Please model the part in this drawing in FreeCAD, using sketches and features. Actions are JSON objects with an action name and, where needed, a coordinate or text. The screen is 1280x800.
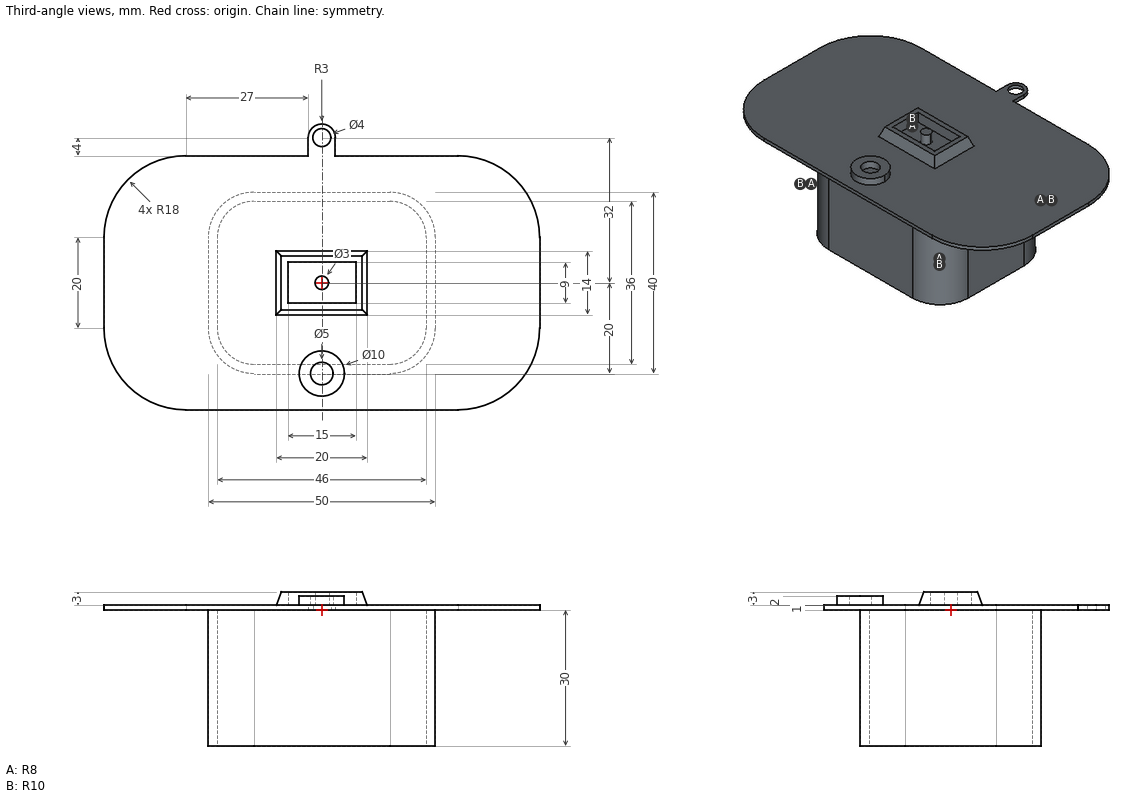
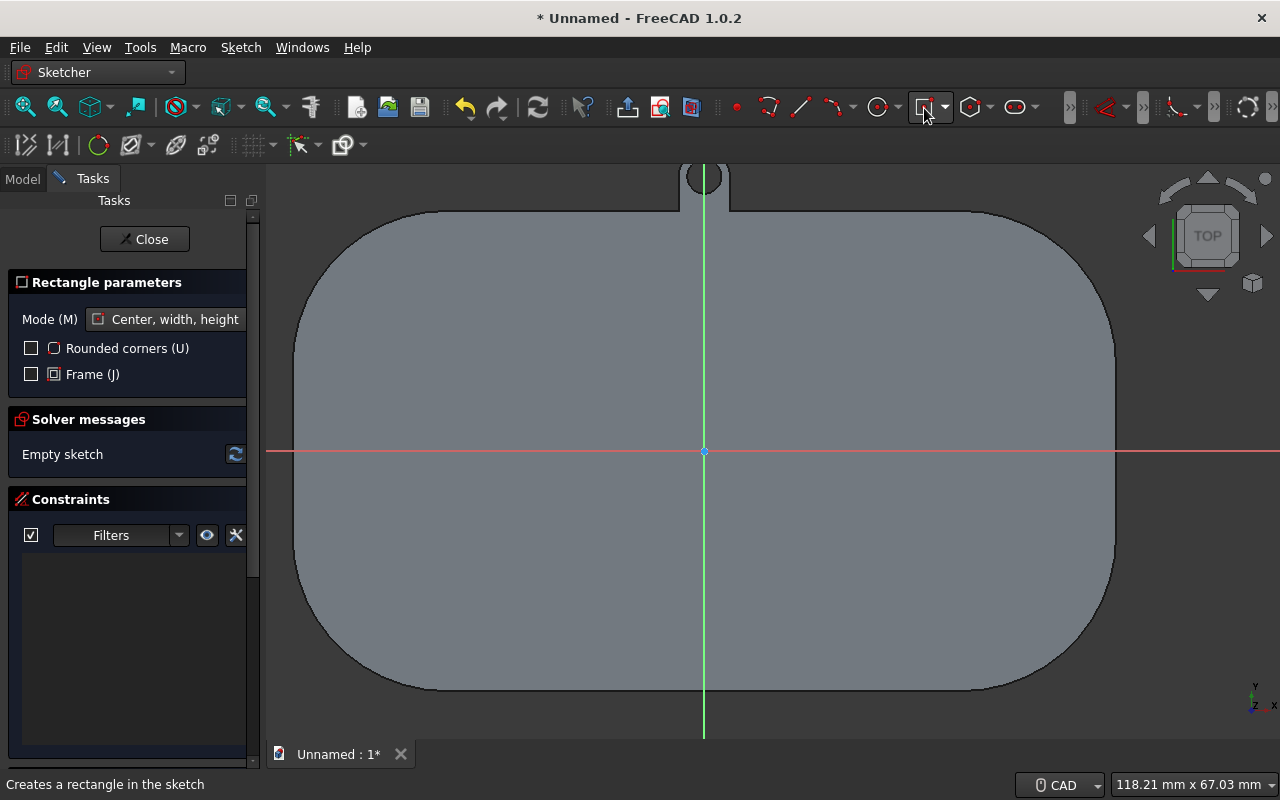
{"action": "left_click", "coordinate": [704, 451]}
{"action": "mouse_move", "coordinate": [919, 279]}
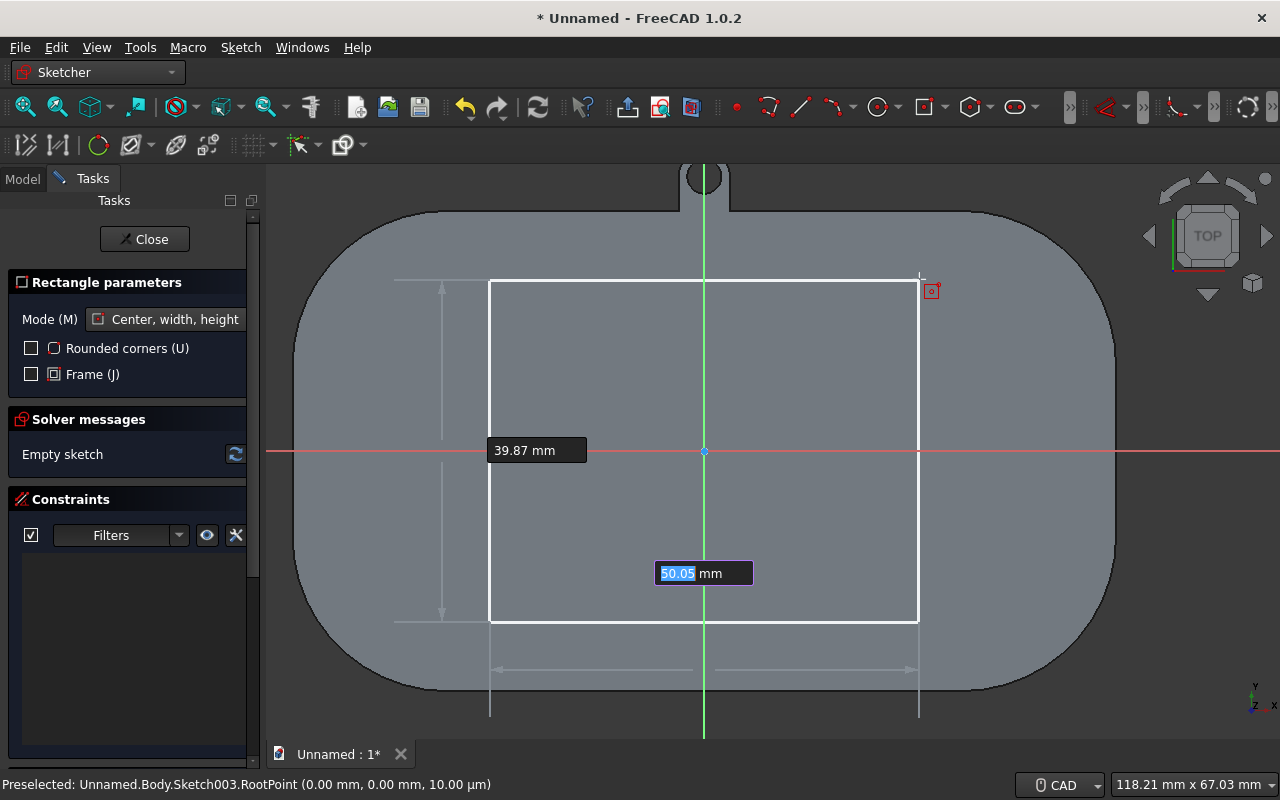
{"action": "type", "text": "50"}
{"action": "key", "text": "Tab"}
{"action": "type", "text": "40"}
{"action": "key", "text": "Return"}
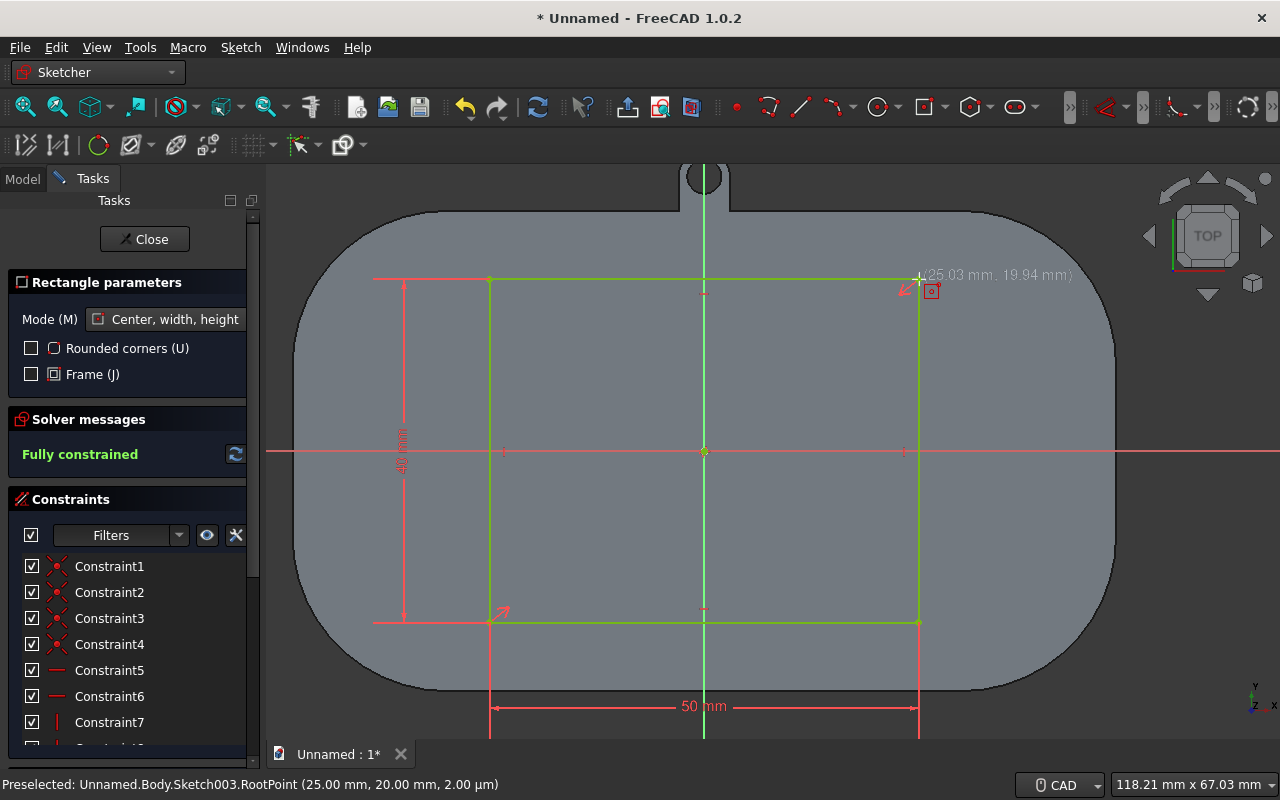
{"action": "left_click", "coordinate": [704, 451]}
{"action": "mouse_move", "coordinate": [902, 297]}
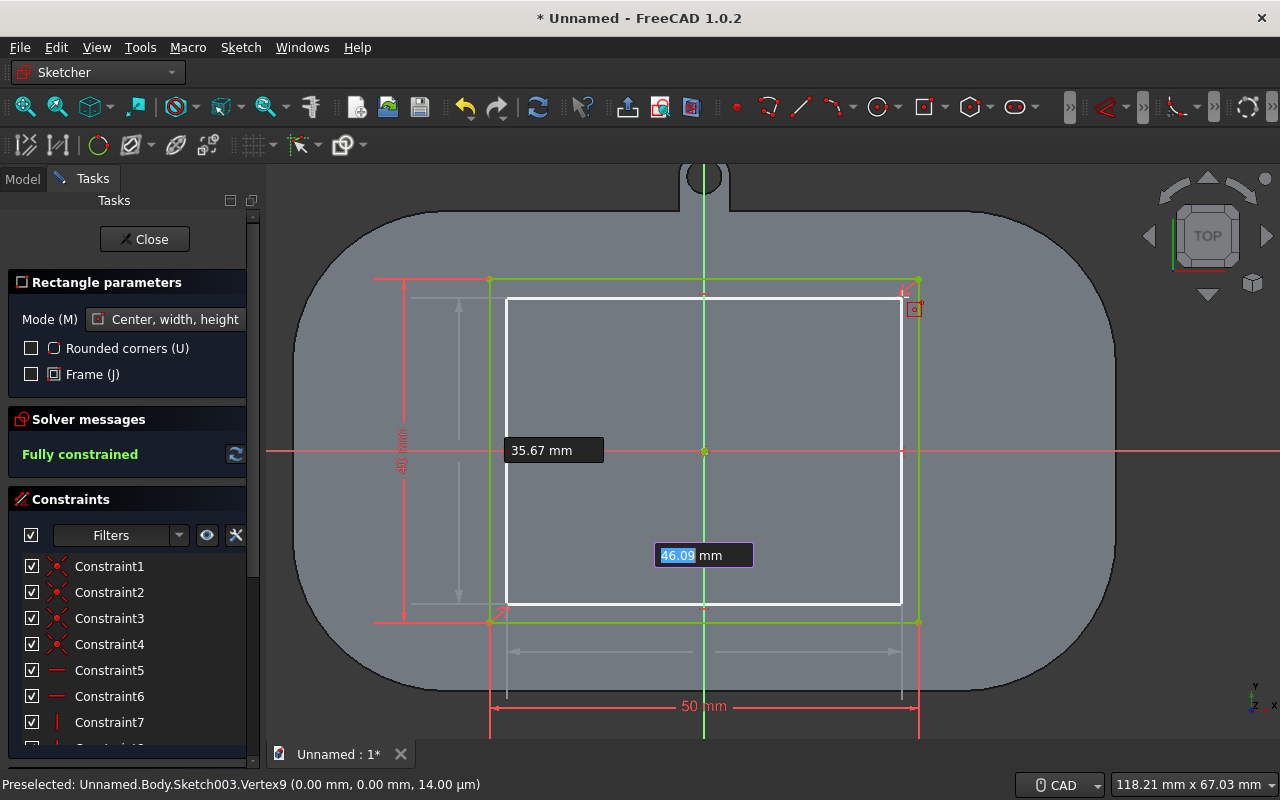
{"action": "type", "text": "46"}
{"action": "key", "text": "Tab"}
{"action": "type", "text": "36"}
{"action": "key", "text": "Return"}
{"action": "key", "text": "Escape"}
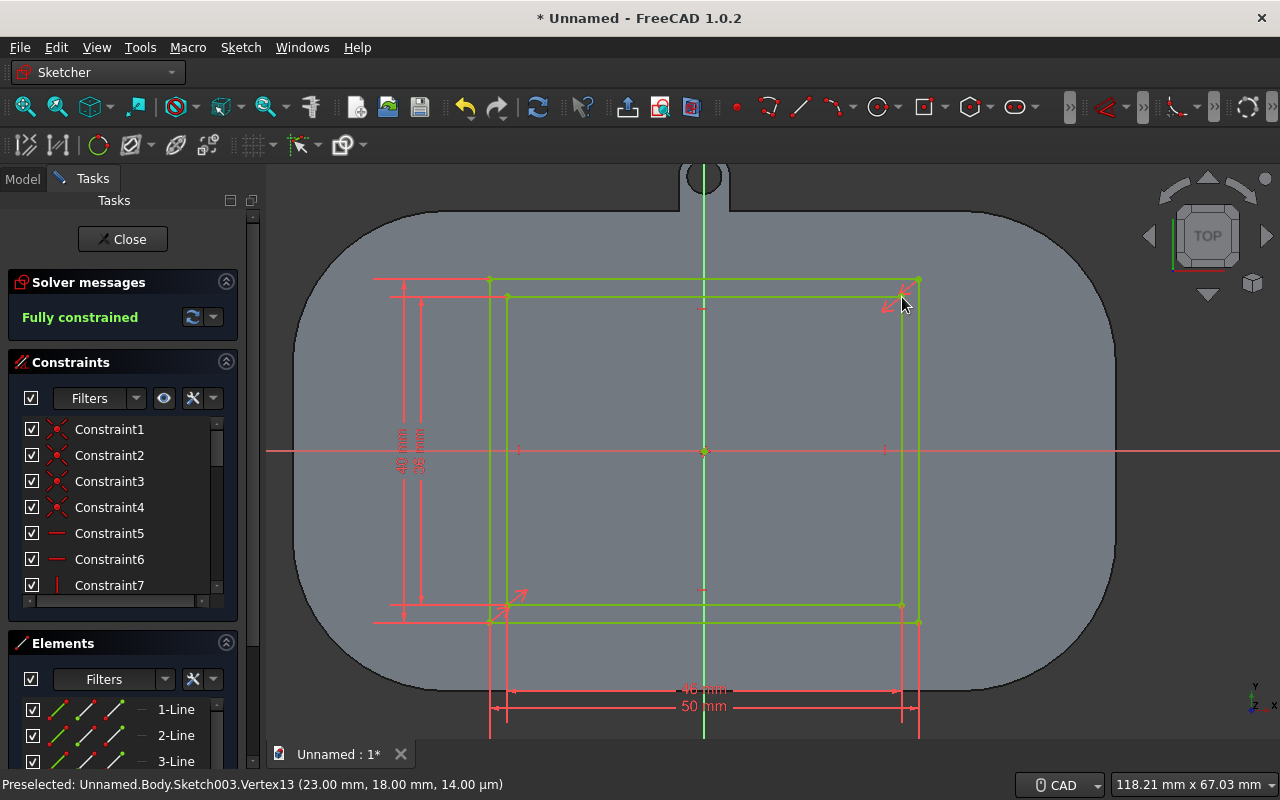
{"action": "left_click", "coordinate": [123, 239]}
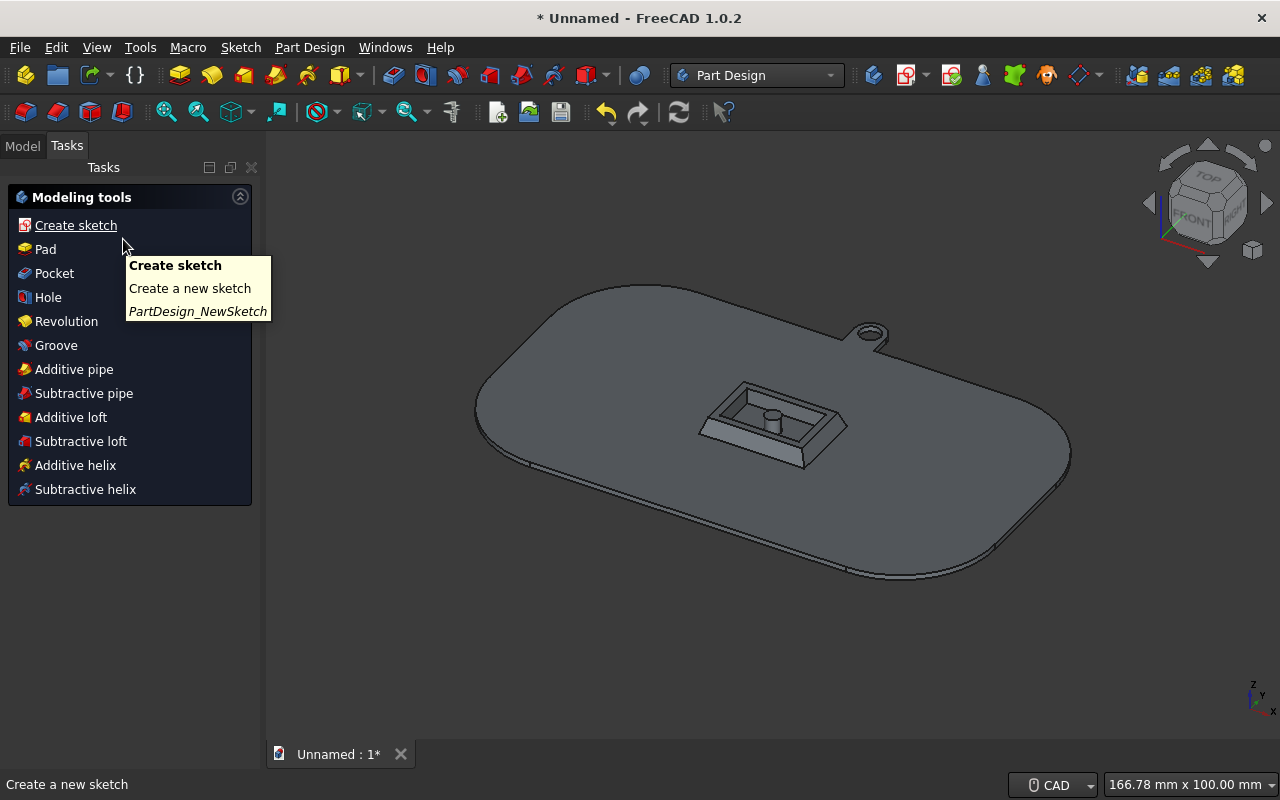
{"action": "left_click", "coordinate": [180, 76]}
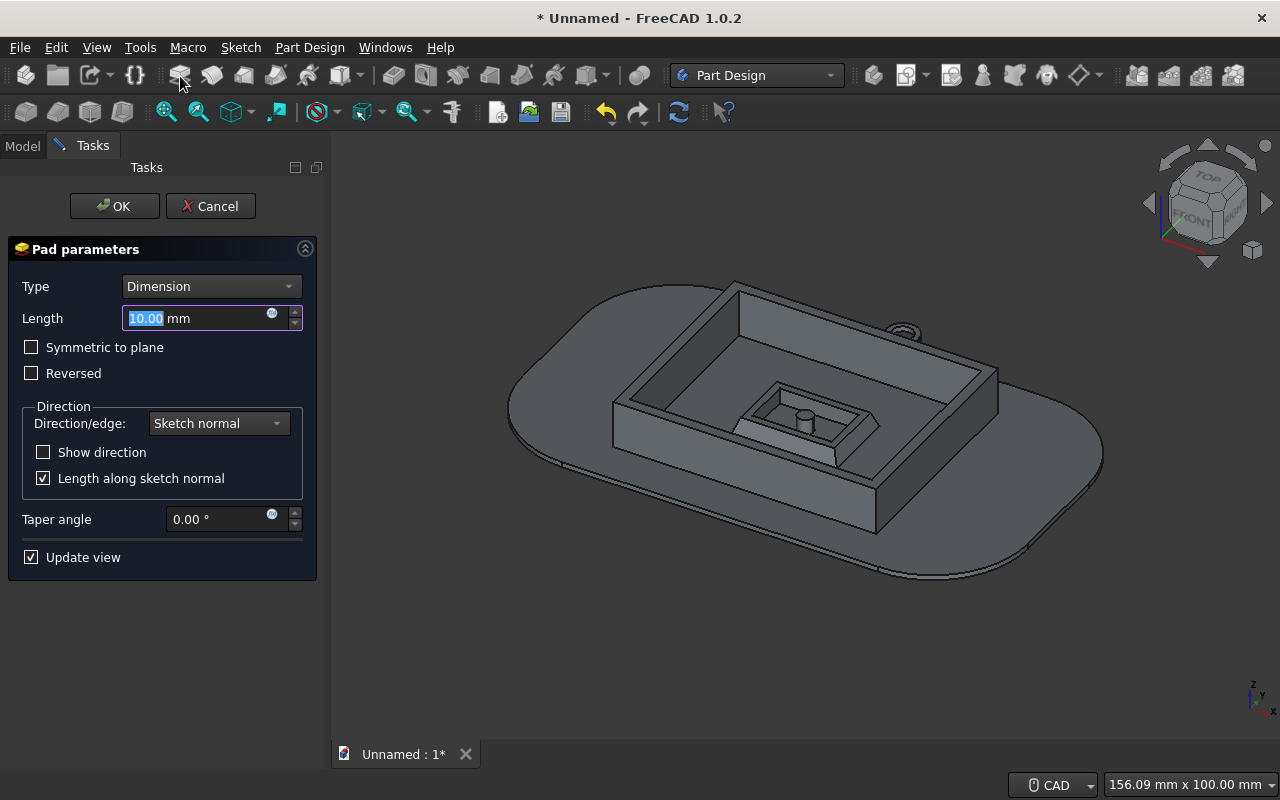
{"action": "type", "text": "30"}
{"action": "key", "text": "Tab"}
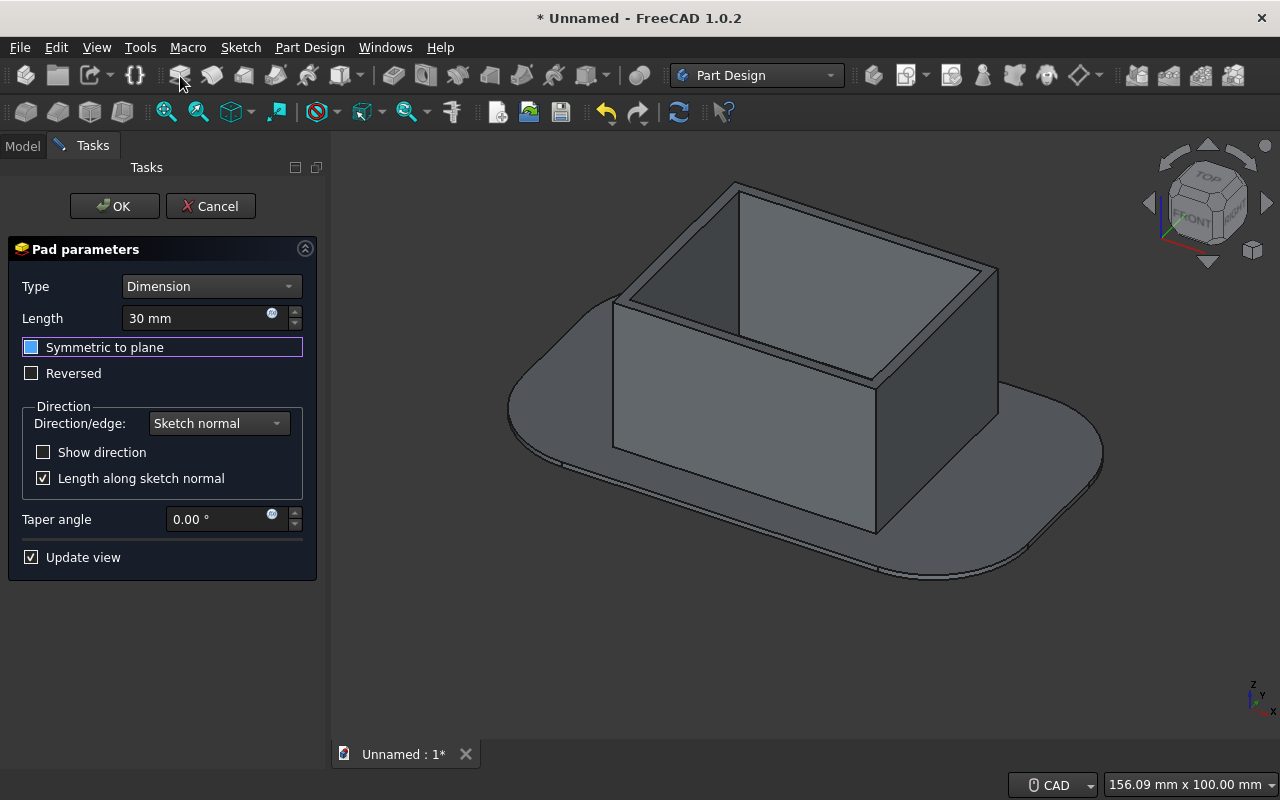
{"action": "left_click", "coordinate": [30, 373]}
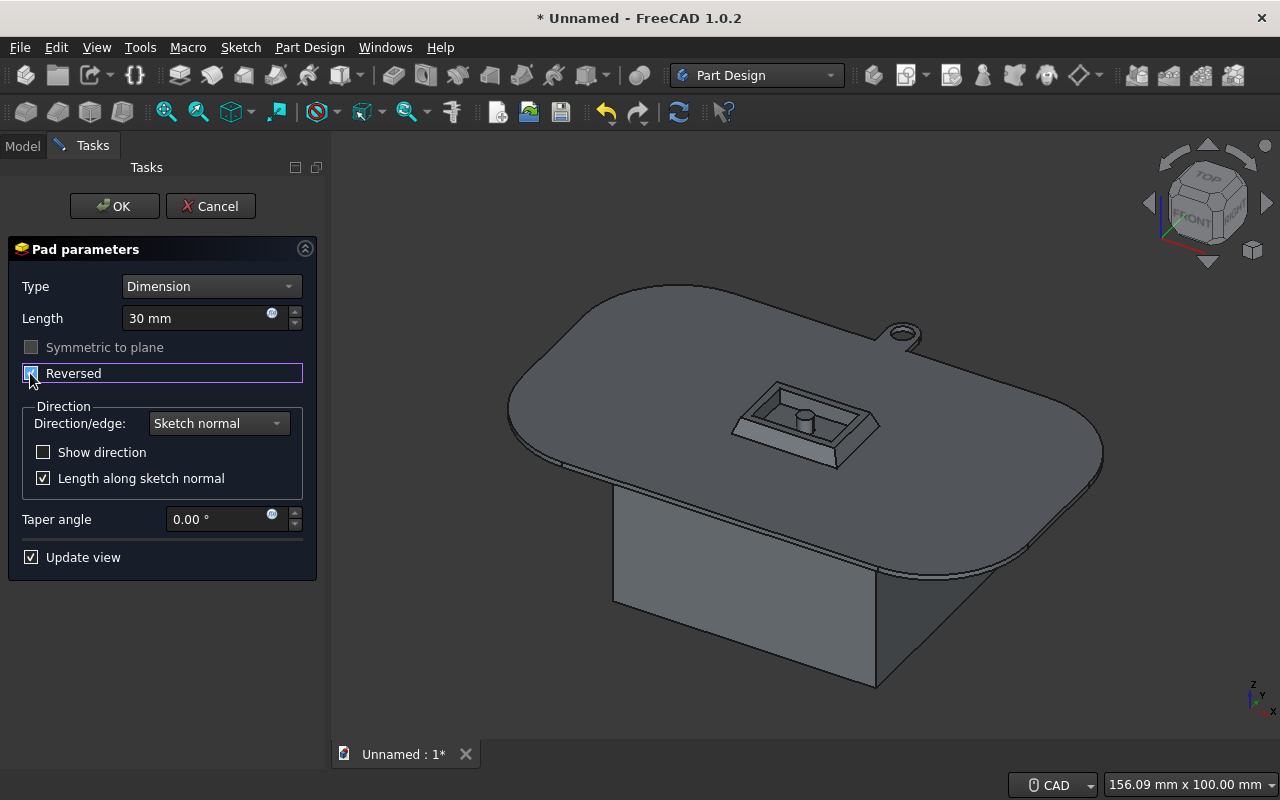
{"action": "left_click", "coordinate": [115, 206]}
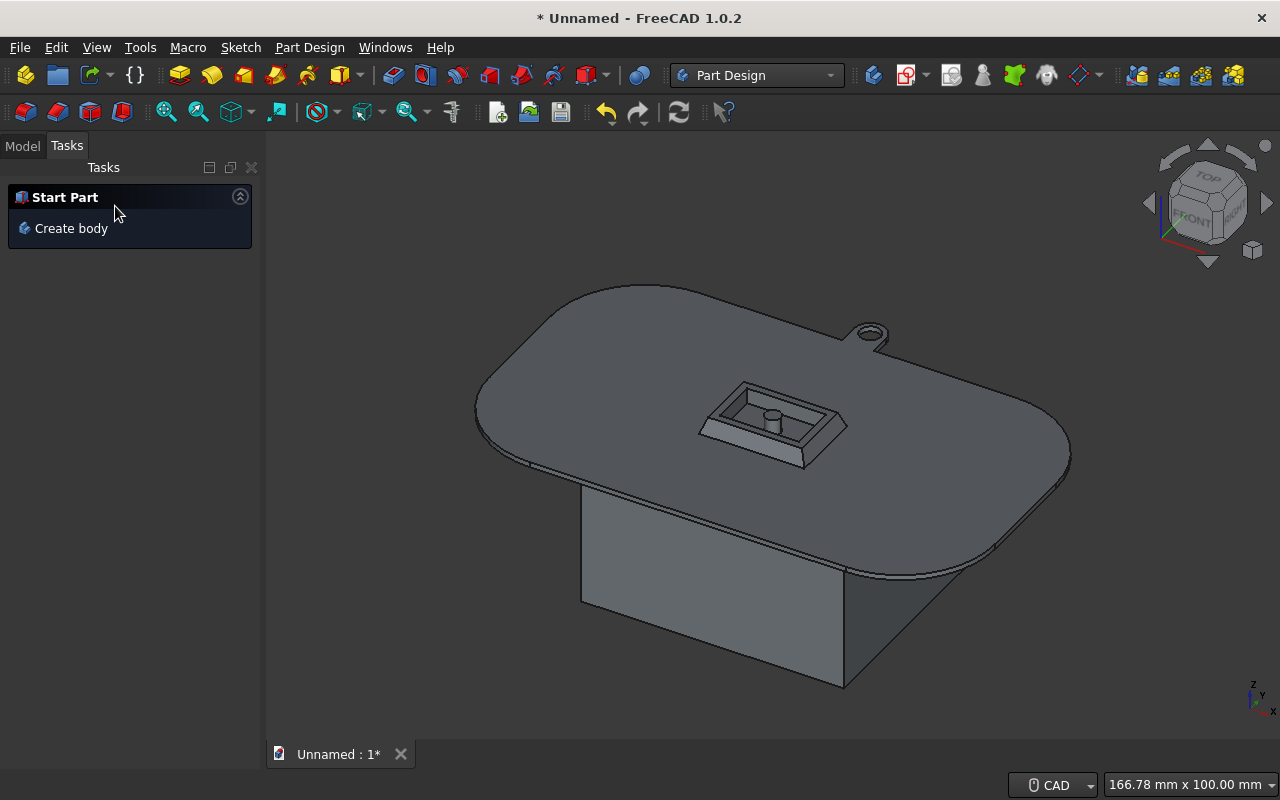
{"action": "left_click", "coordinate": [168, 112]}